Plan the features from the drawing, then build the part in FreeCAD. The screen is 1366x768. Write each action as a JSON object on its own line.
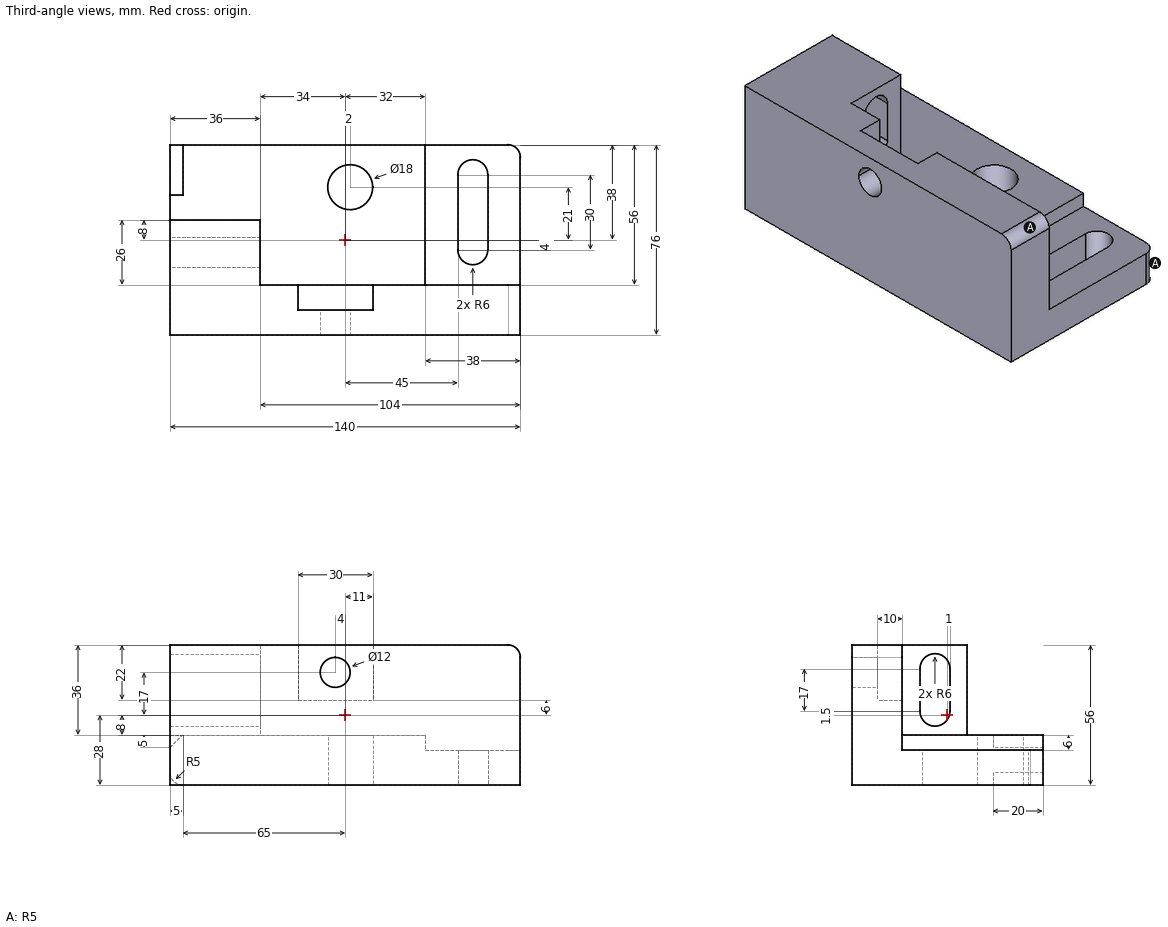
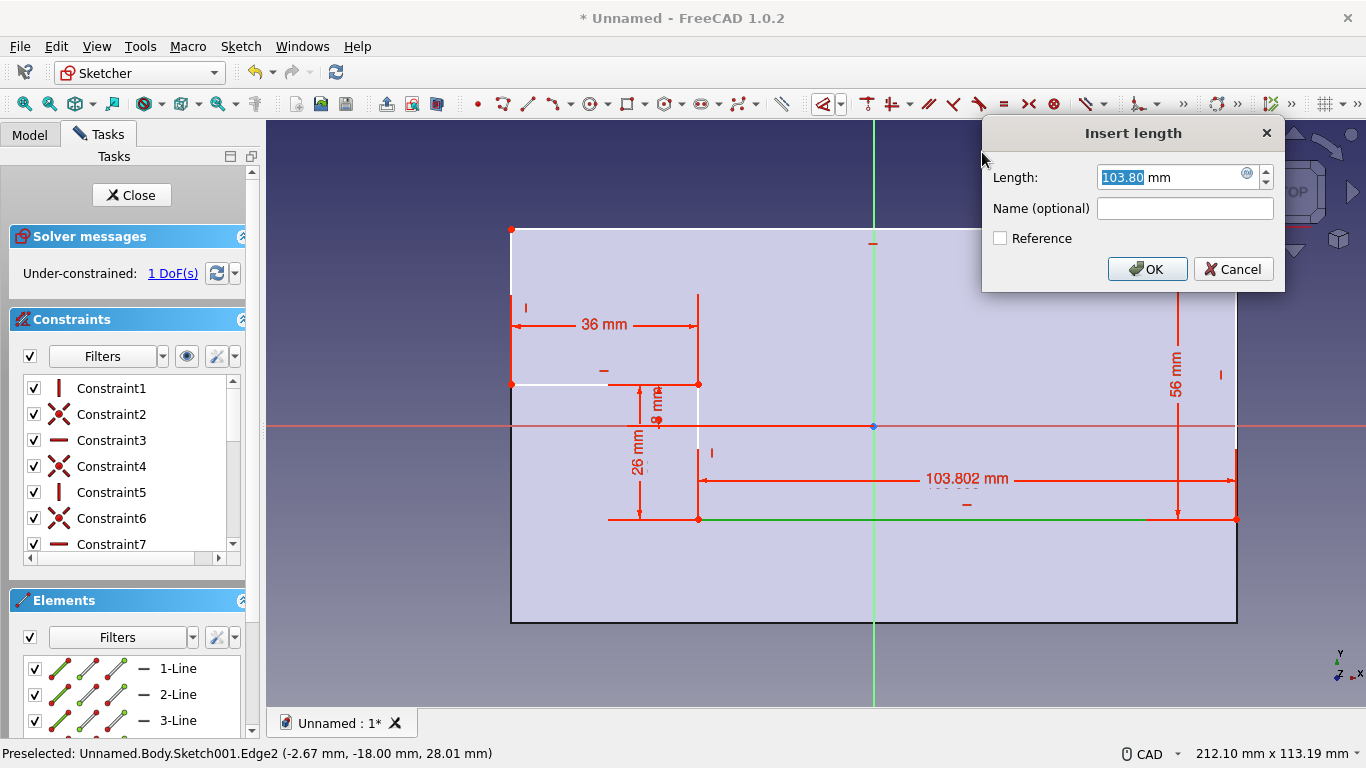
{"action": "type", "text": "104"}
{"action": "key", "text": "Return"}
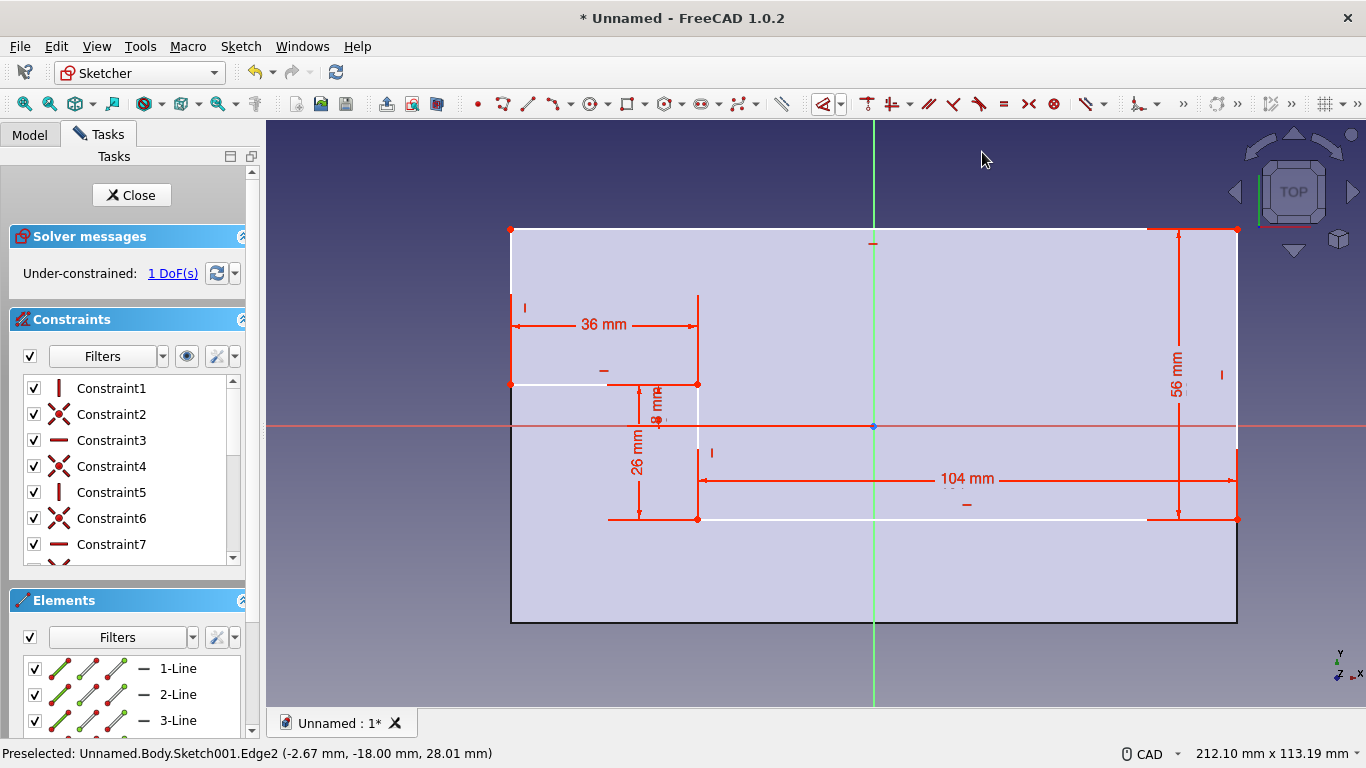
{"action": "left_click", "coordinate": [698, 385]}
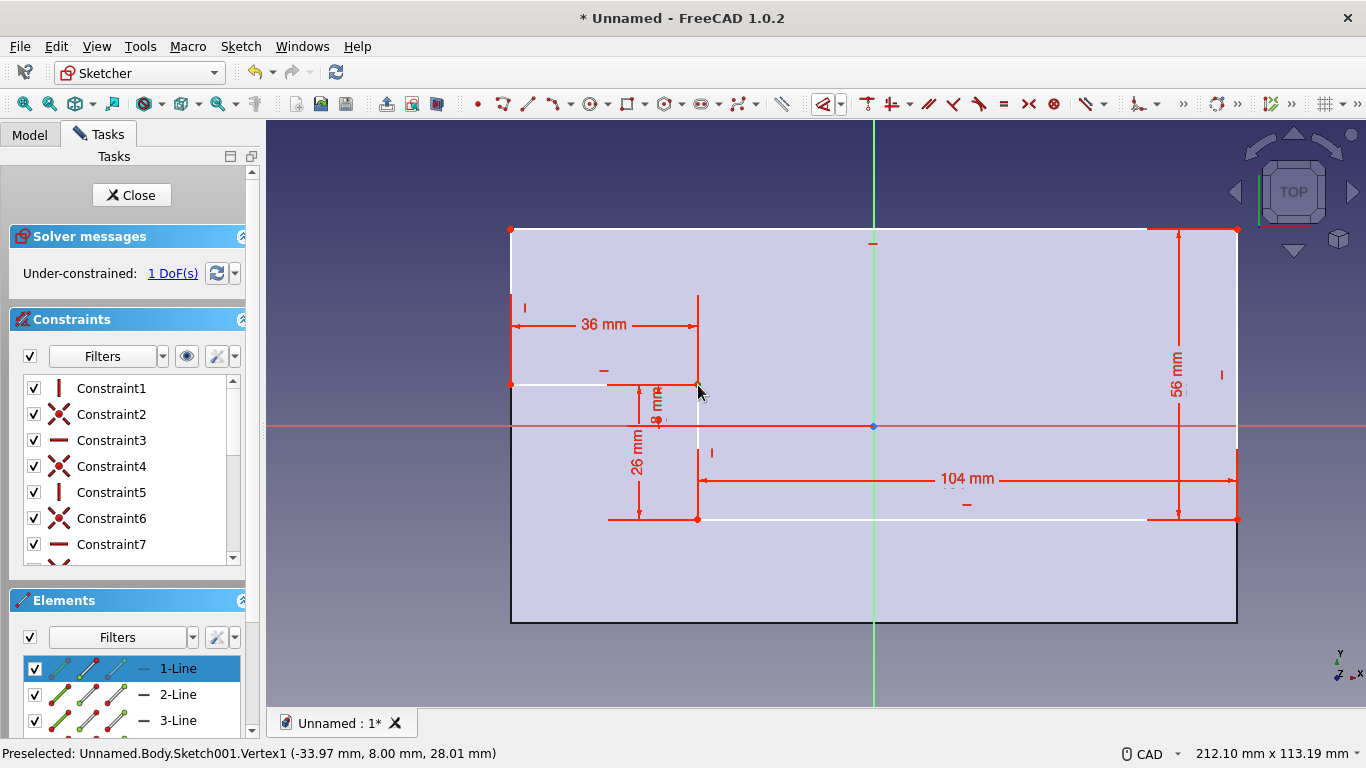
{"action": "left_click", "coordinate": [840, 104]}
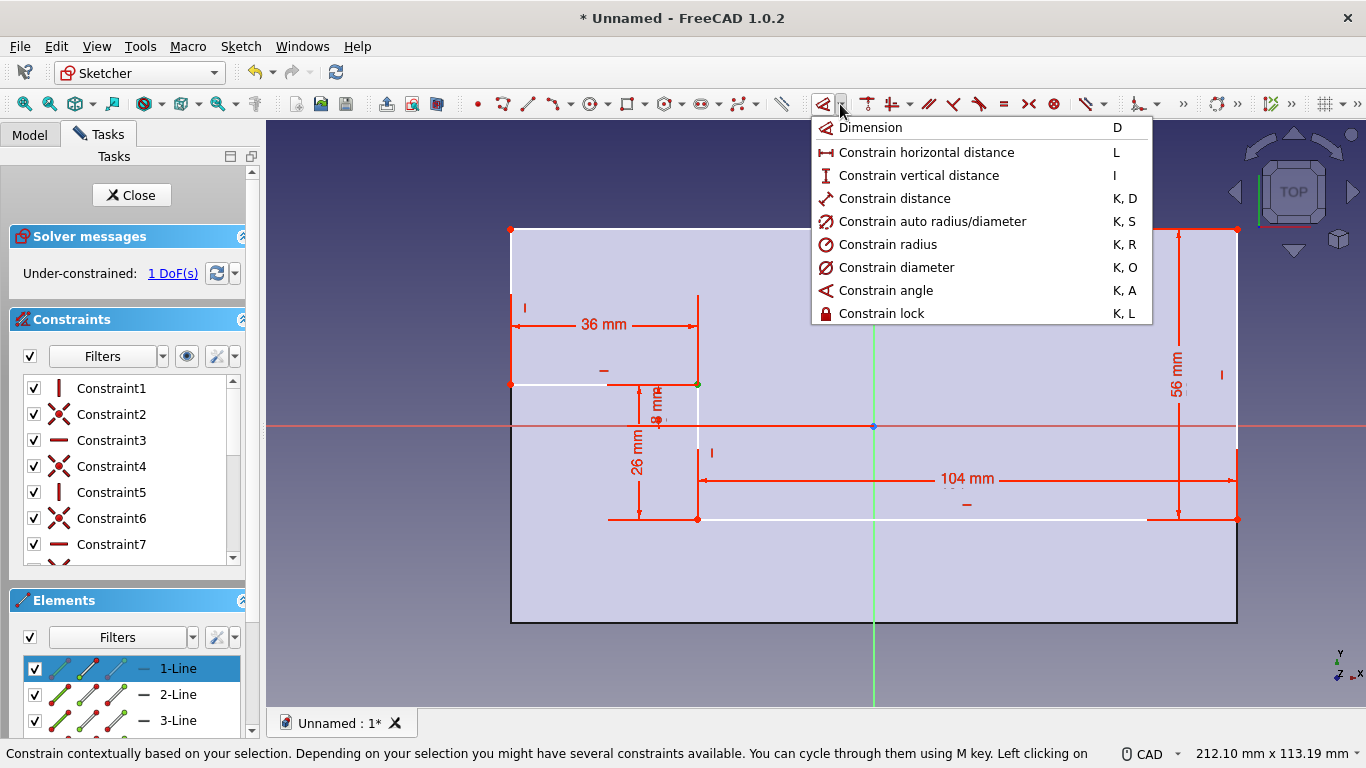
{"action": "left_click", "coordinate": [982, 152]}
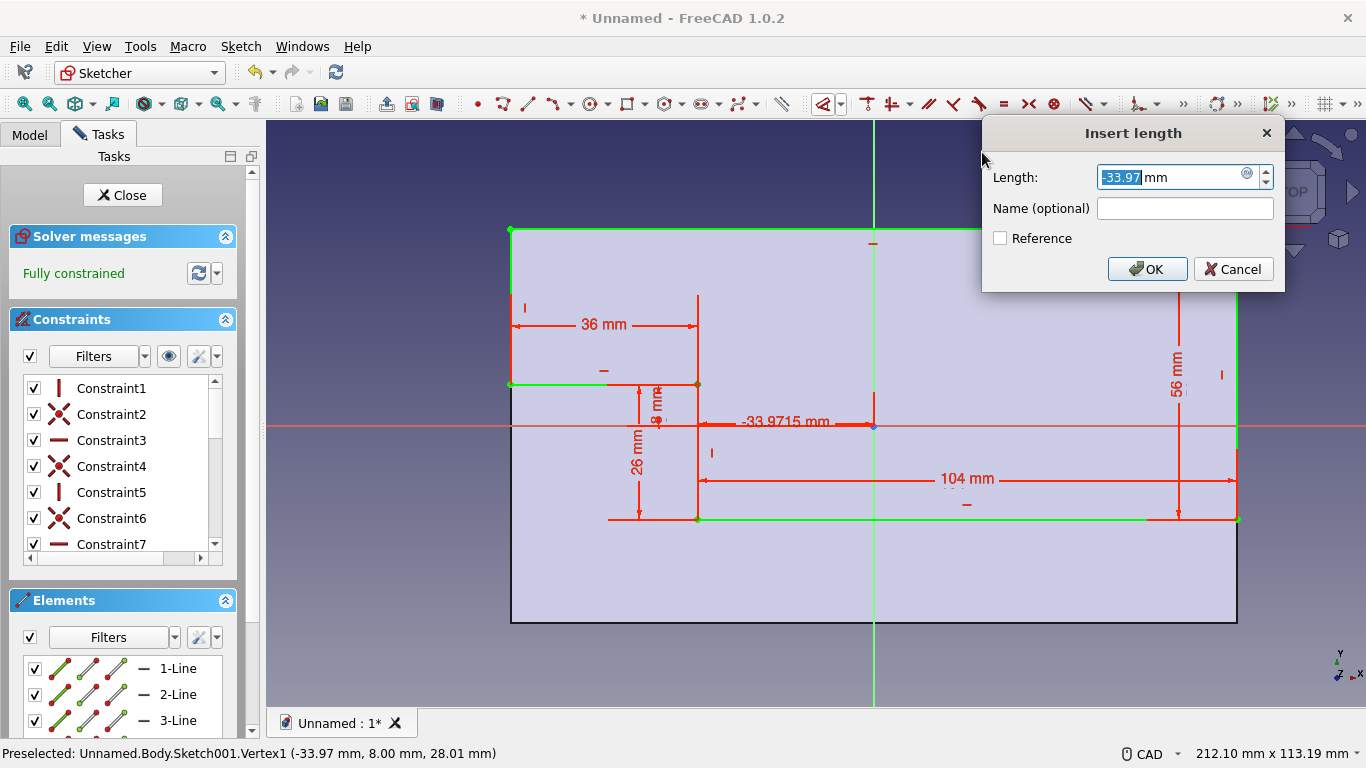
{"action": "type", "text": "-34"}
{"action": "key", "text": "Return"}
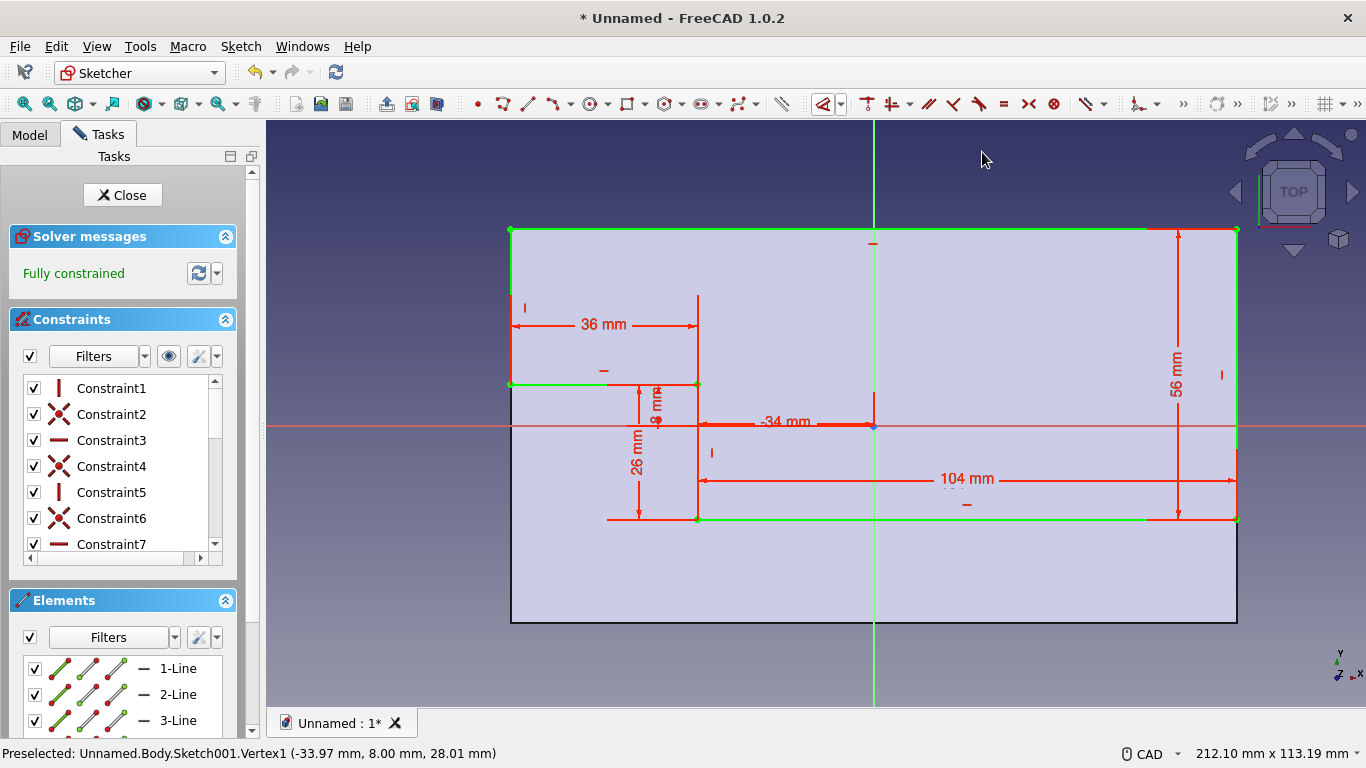
{"action": "left_click", "coordinate": [123, 195]}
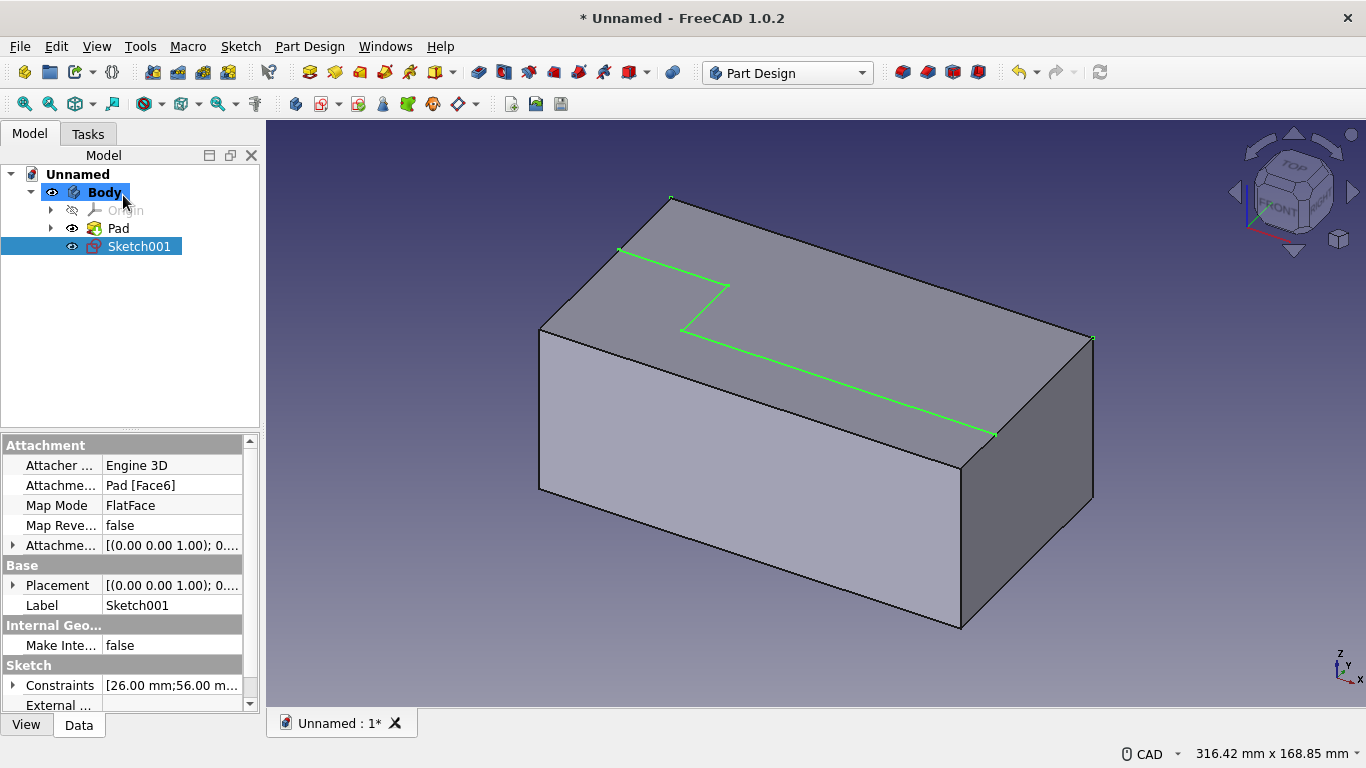
{"action": "left_click", "coordinate": [479, 72]}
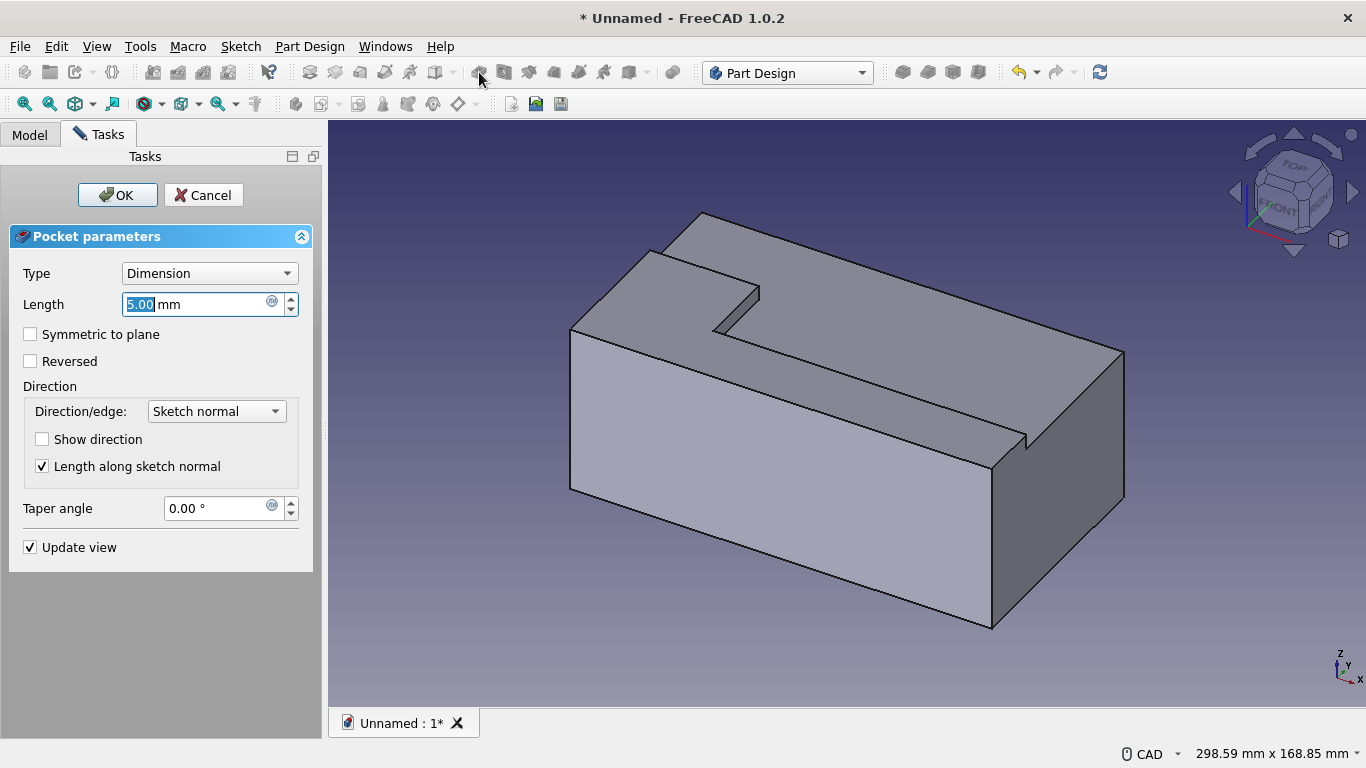
{"action": "type", "text": "36"}
{"action": "key", "text": "Tab"}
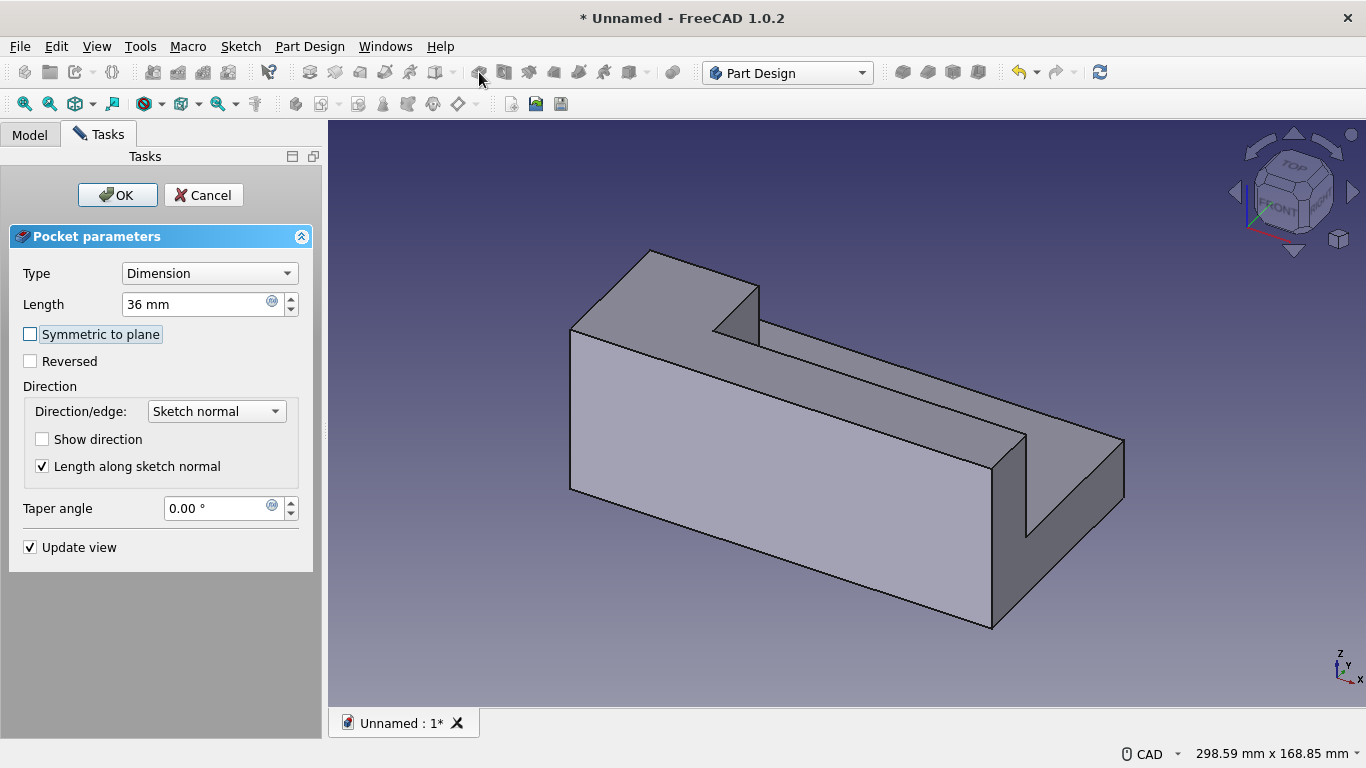
{"action": "left_click", "coordinate": [118, 195]}